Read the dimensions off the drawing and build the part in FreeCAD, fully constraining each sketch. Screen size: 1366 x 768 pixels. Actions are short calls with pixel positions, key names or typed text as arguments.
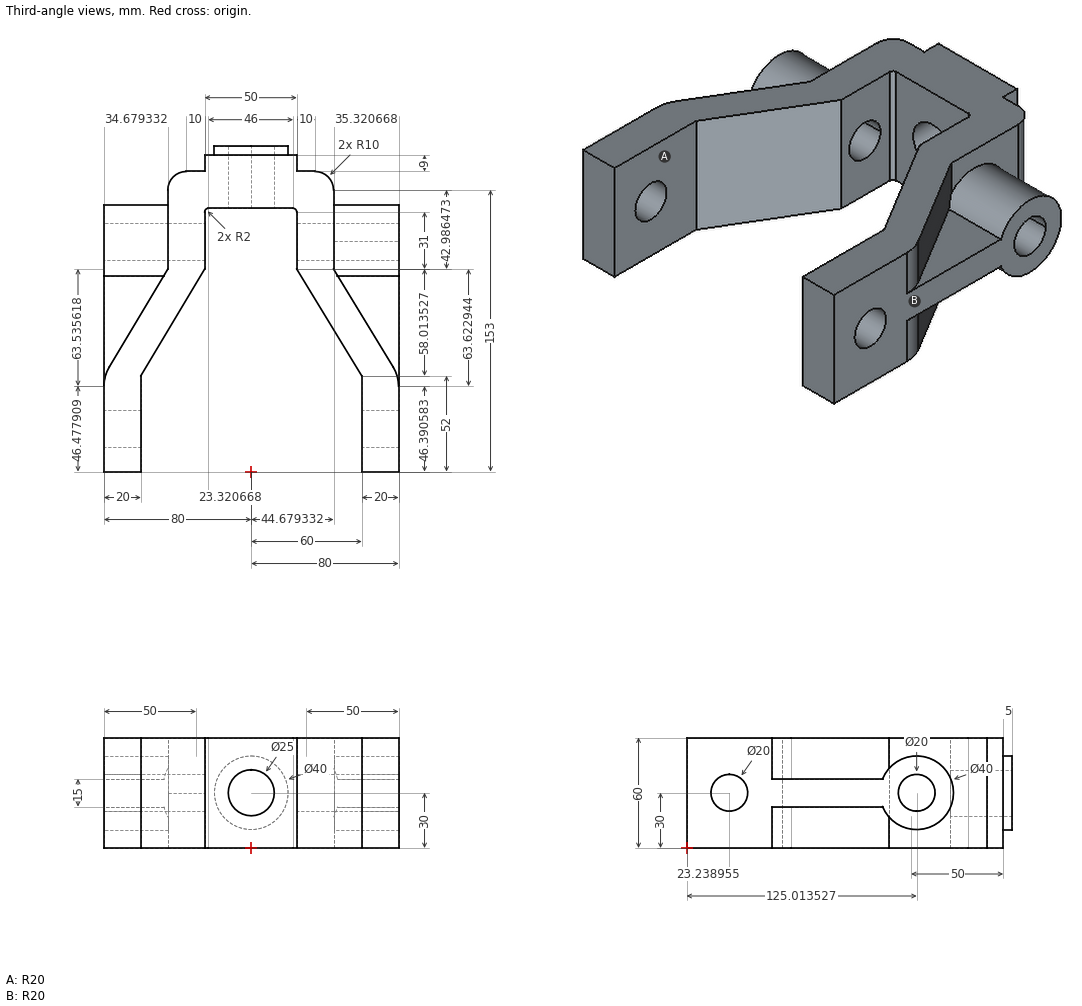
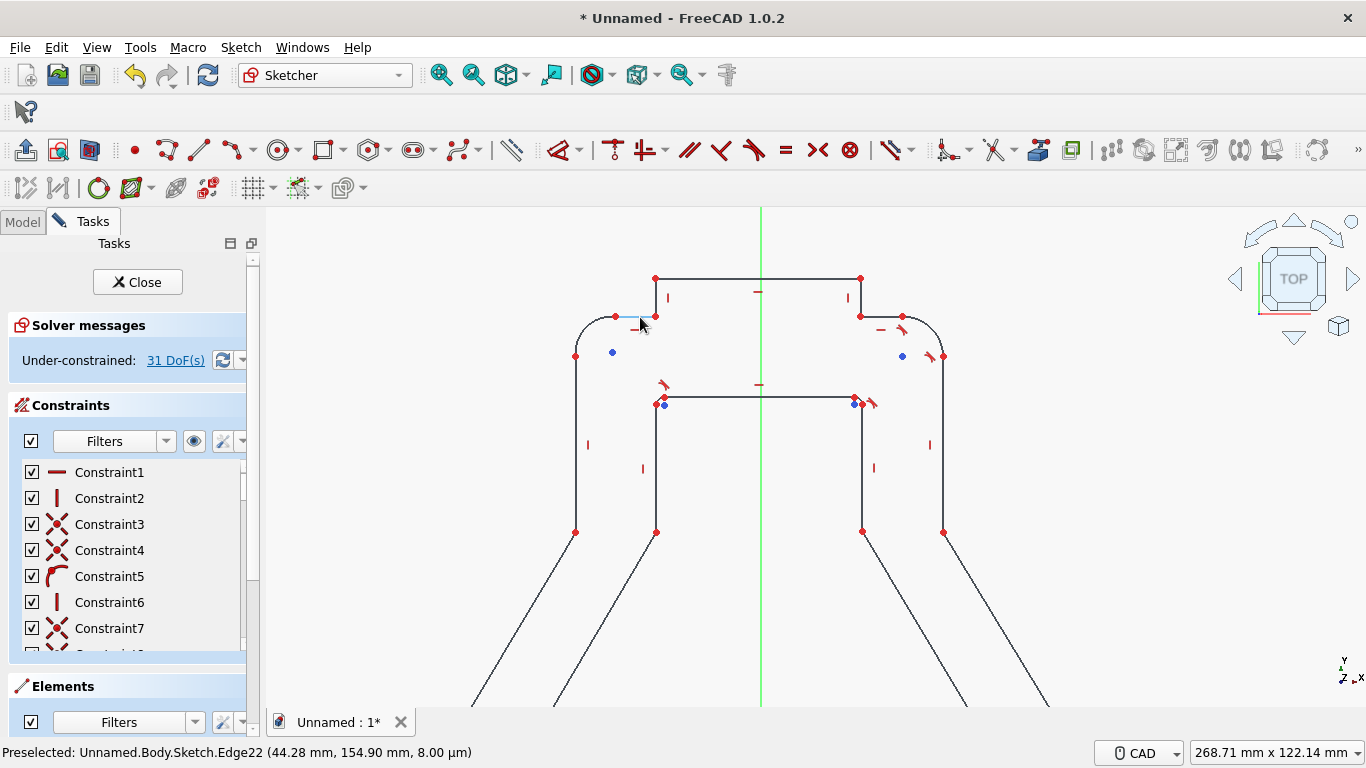
click(640, 317)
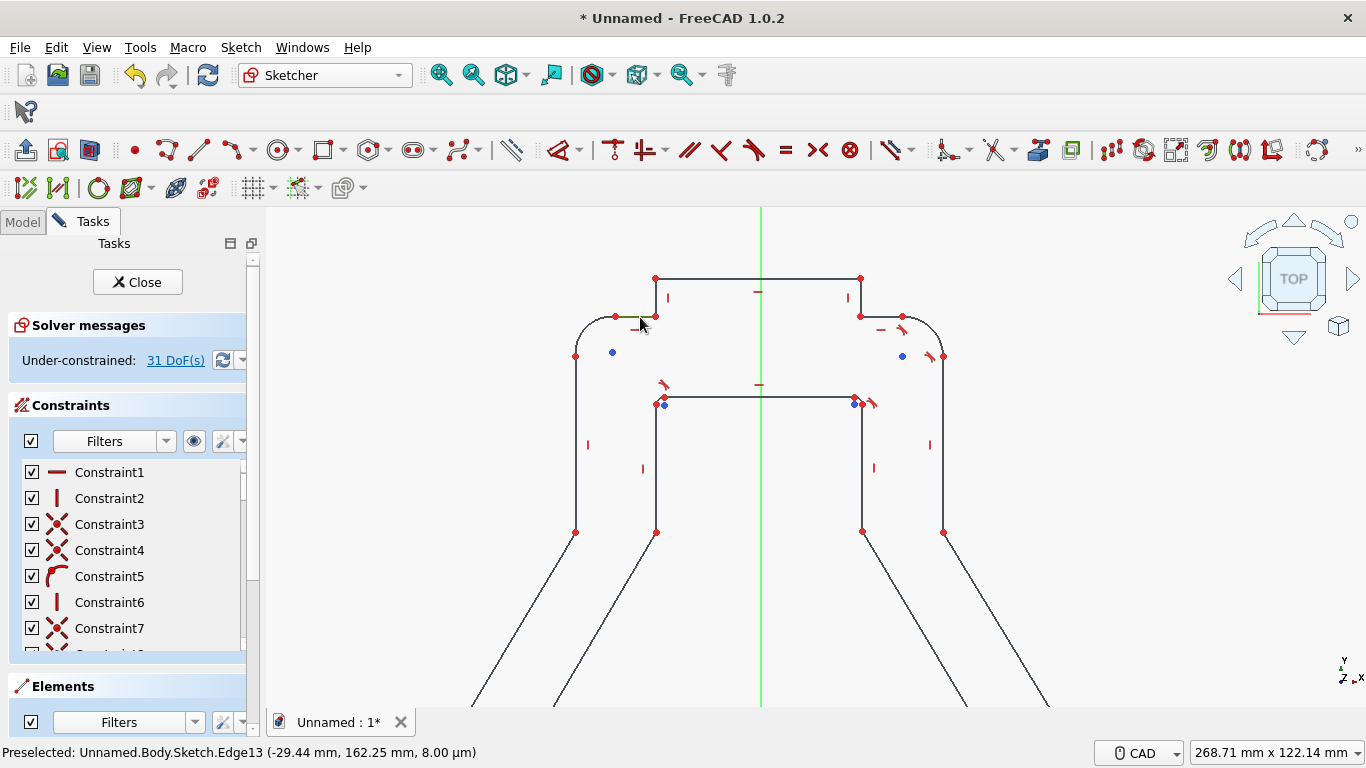
click(597, 320)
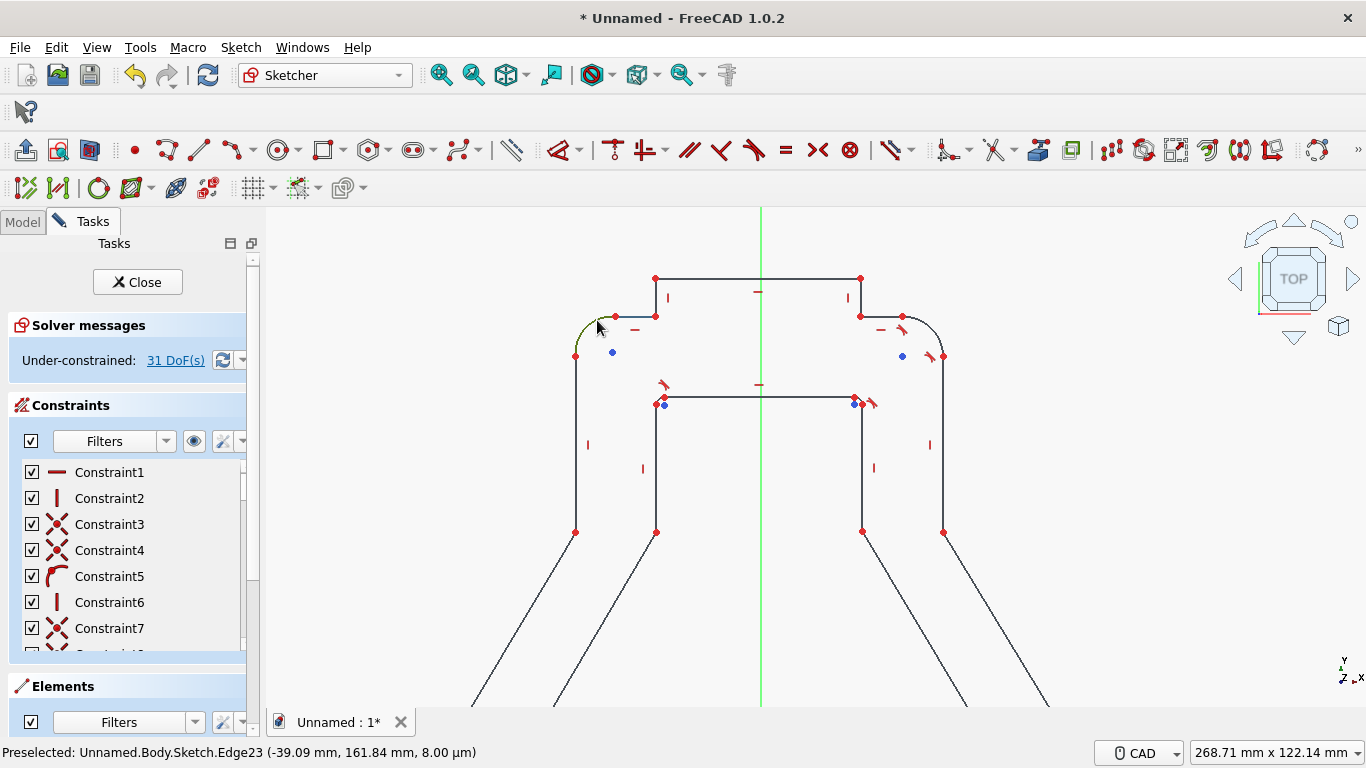
key(t)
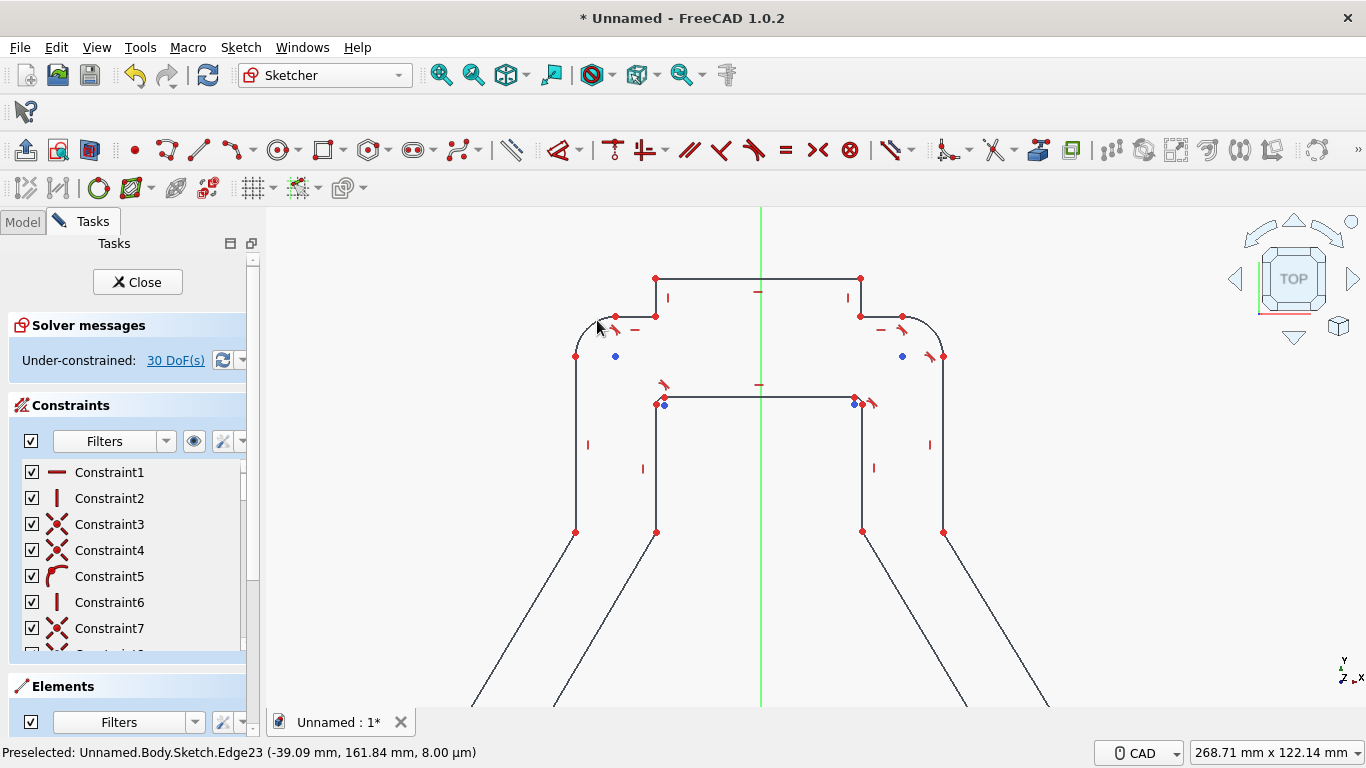
click(576, 410)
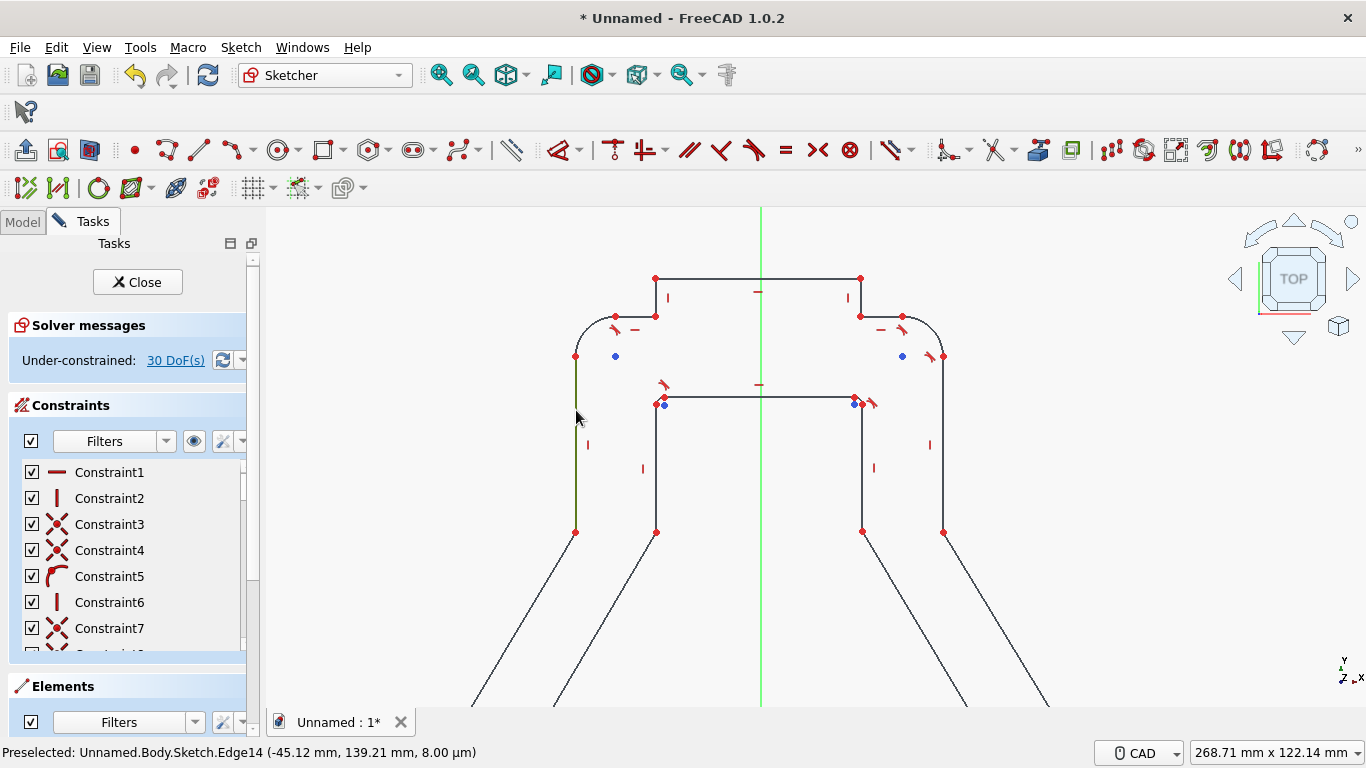
click(598, 321)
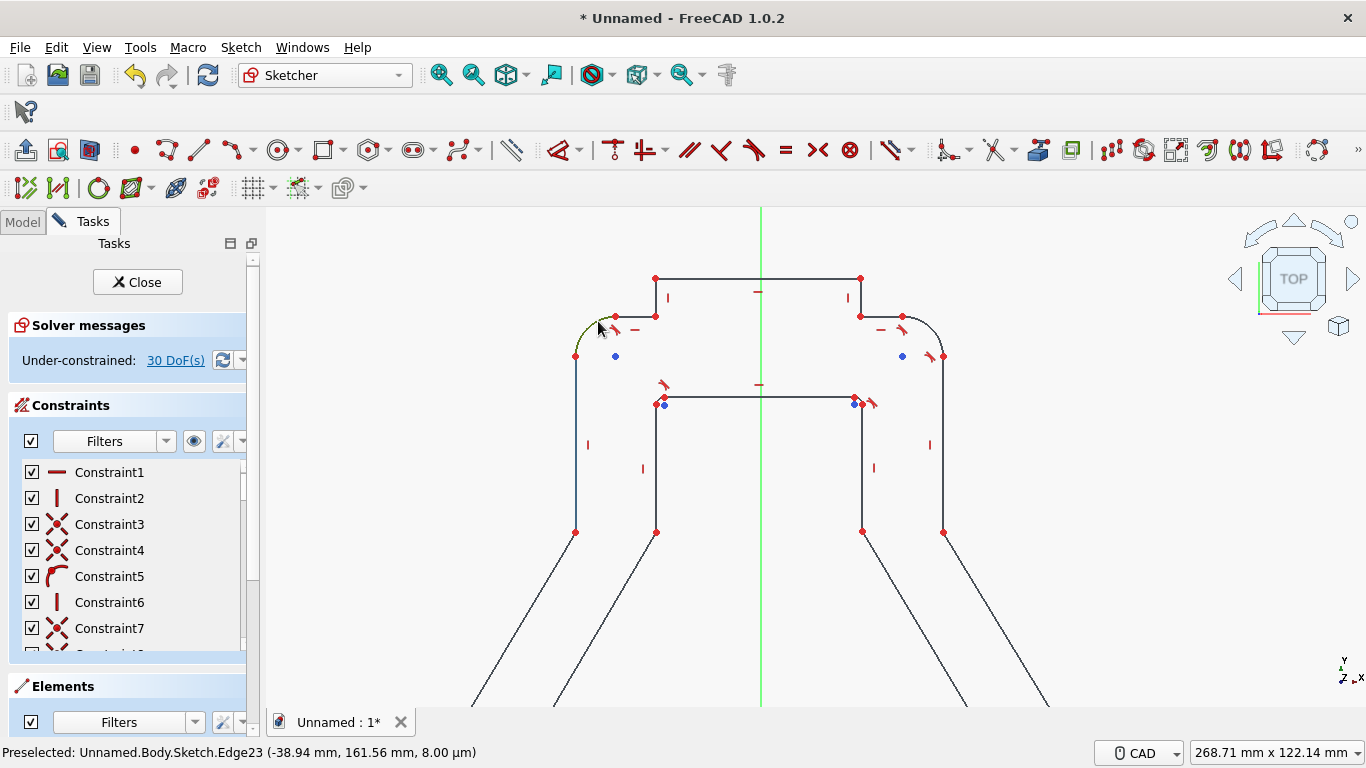
key(t)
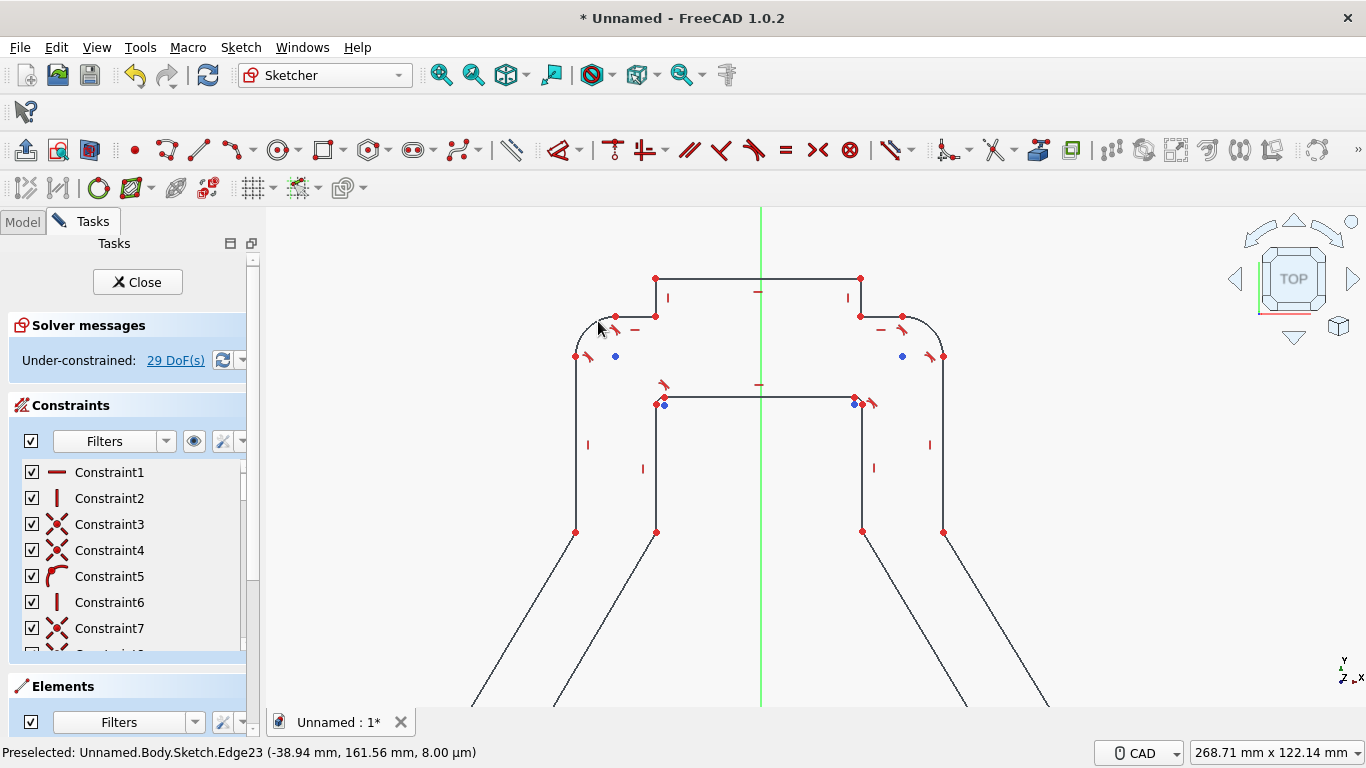
click(656, 494)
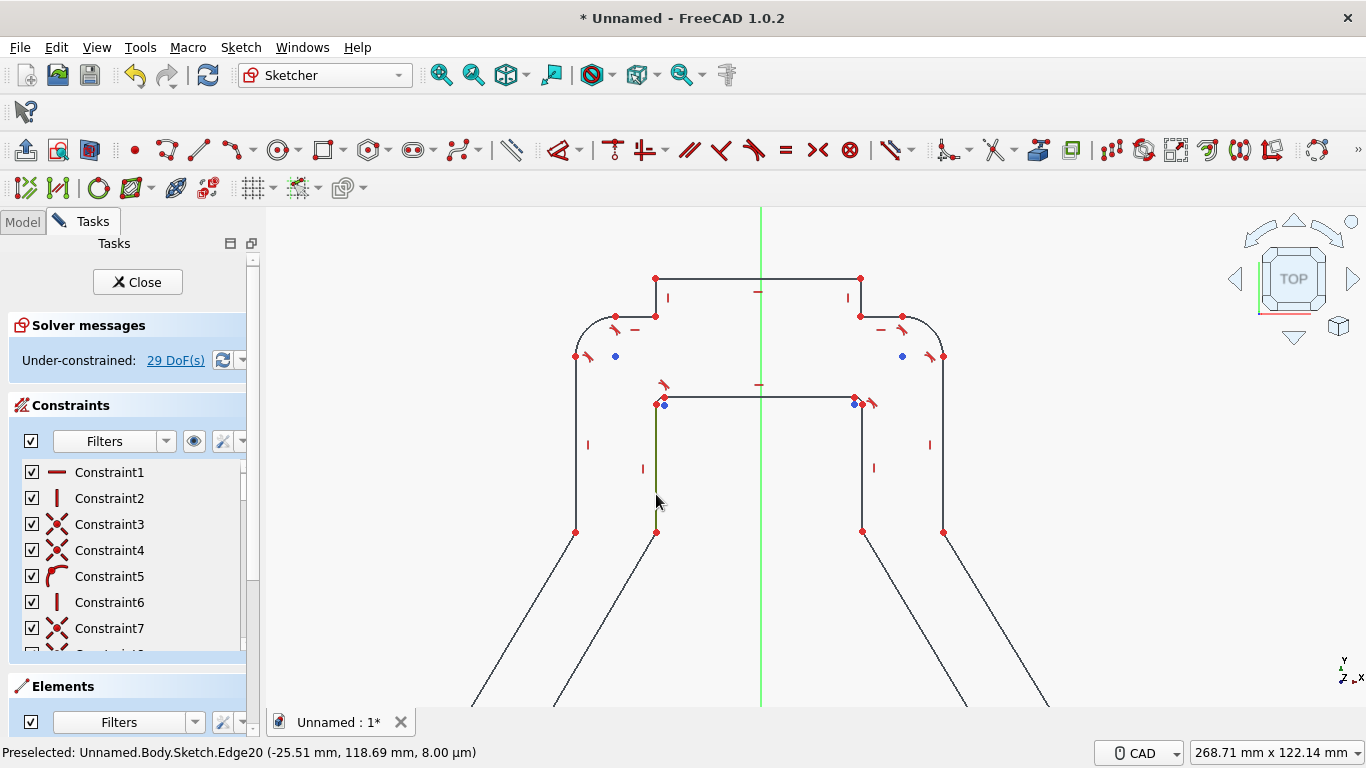
scroll(659, 399, up, 5)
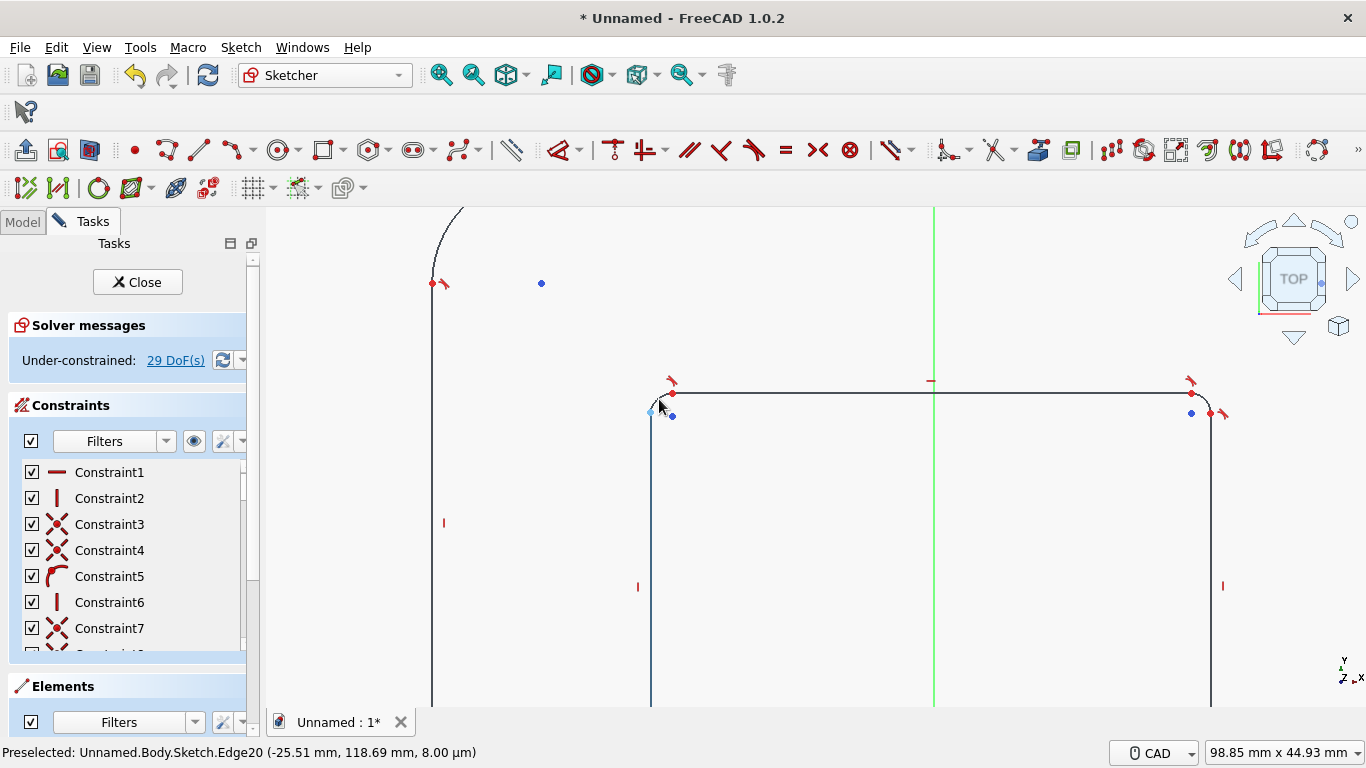
click(658, 399)